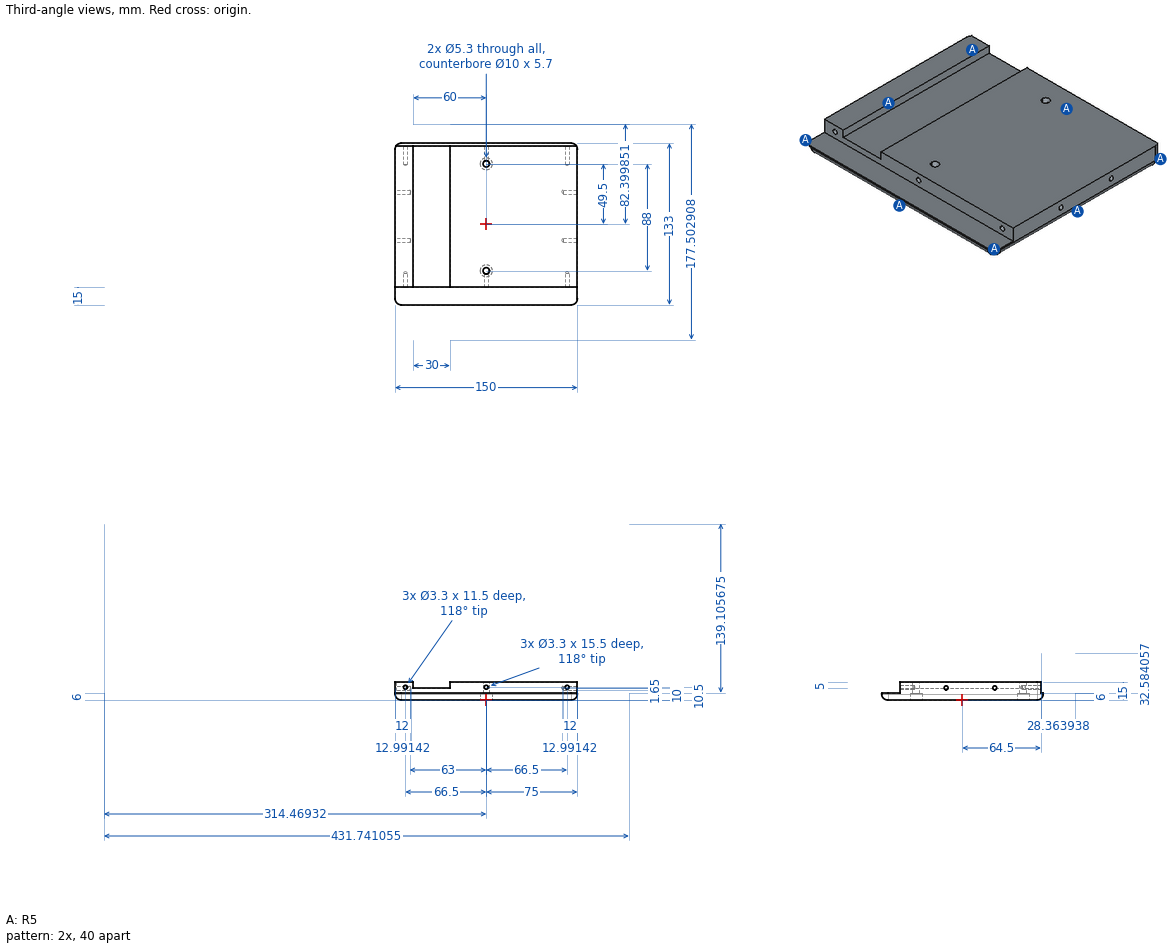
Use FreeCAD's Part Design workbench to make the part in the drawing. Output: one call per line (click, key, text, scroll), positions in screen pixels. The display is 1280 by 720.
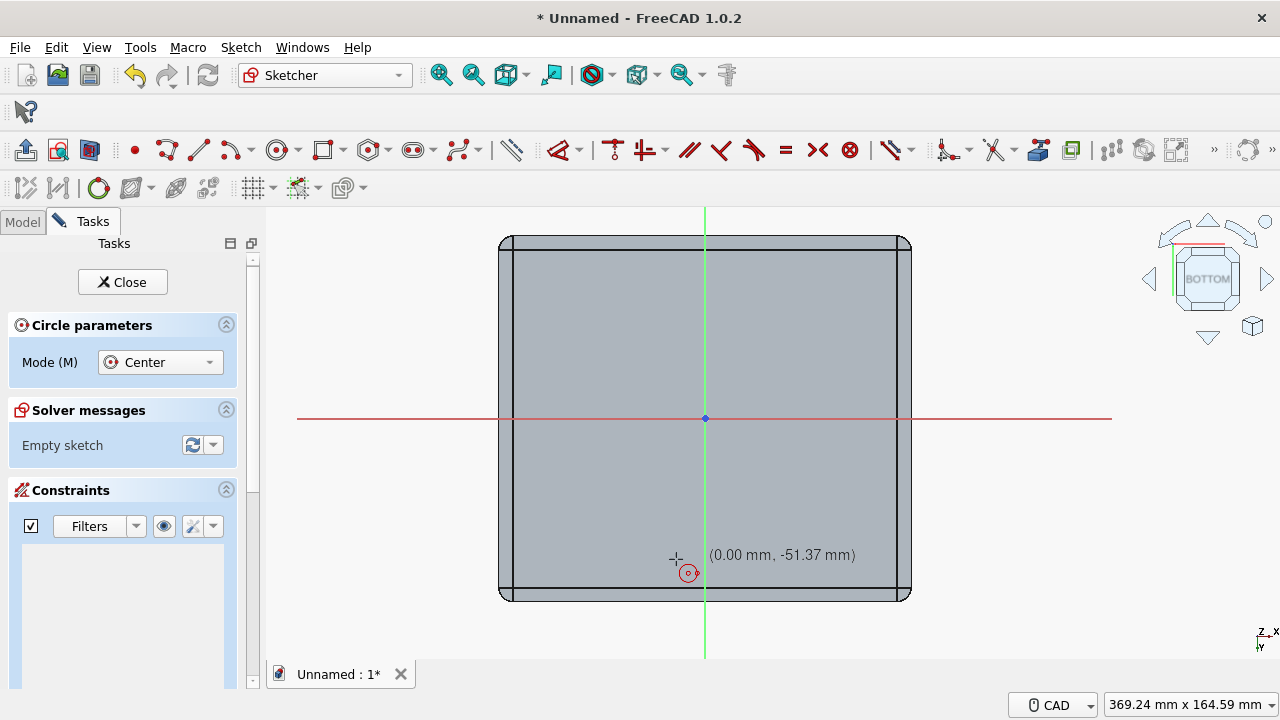
click(705, 555)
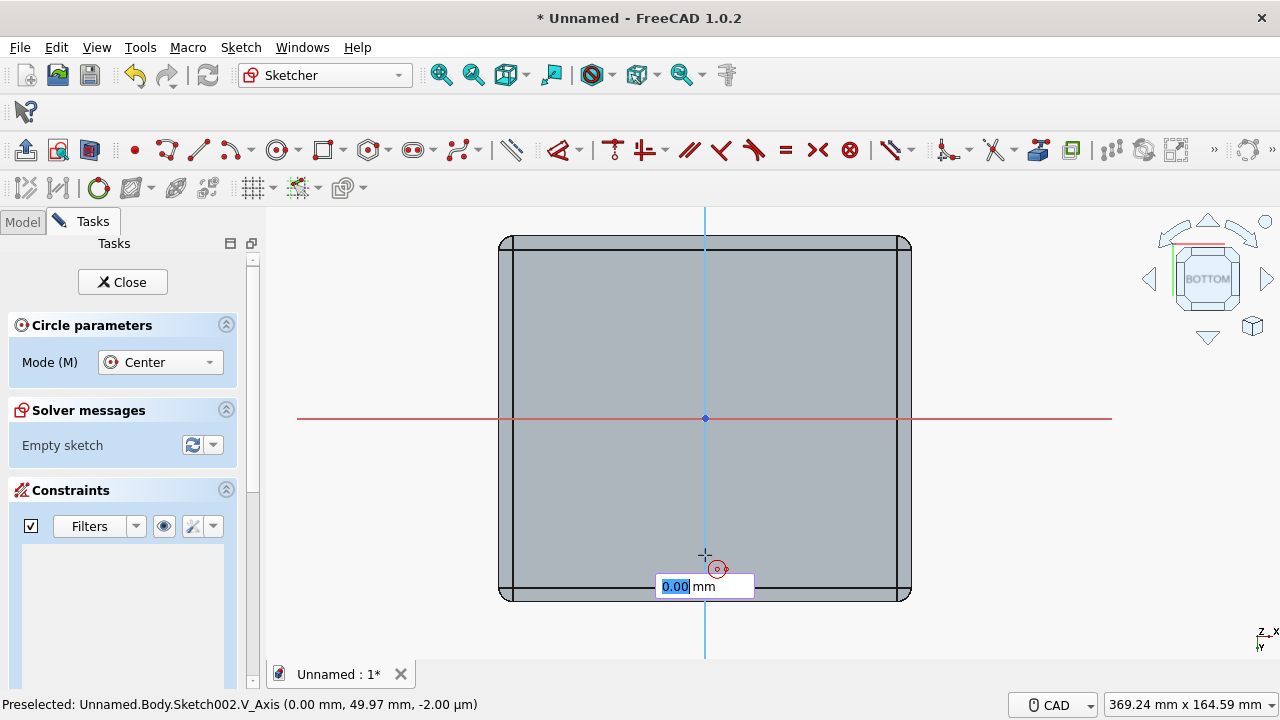
scroll(712, 552, up, 5)
move(711, 551)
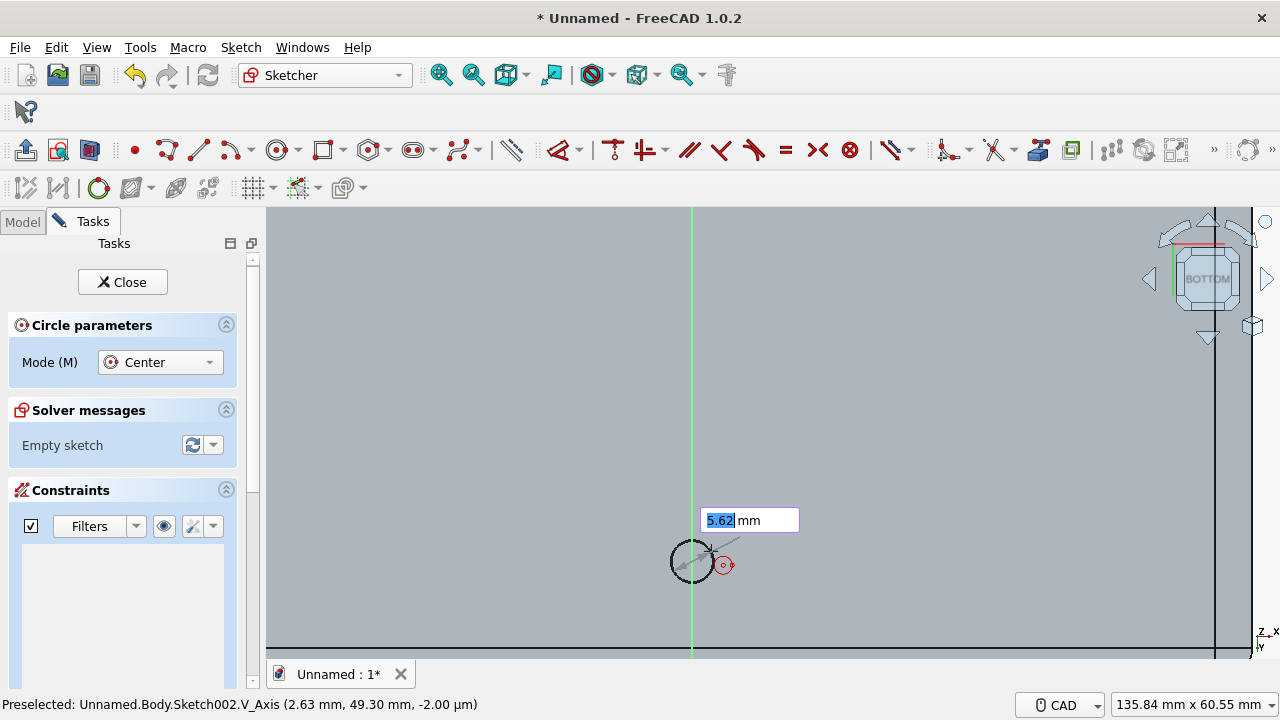
text(5.3)
key(Return)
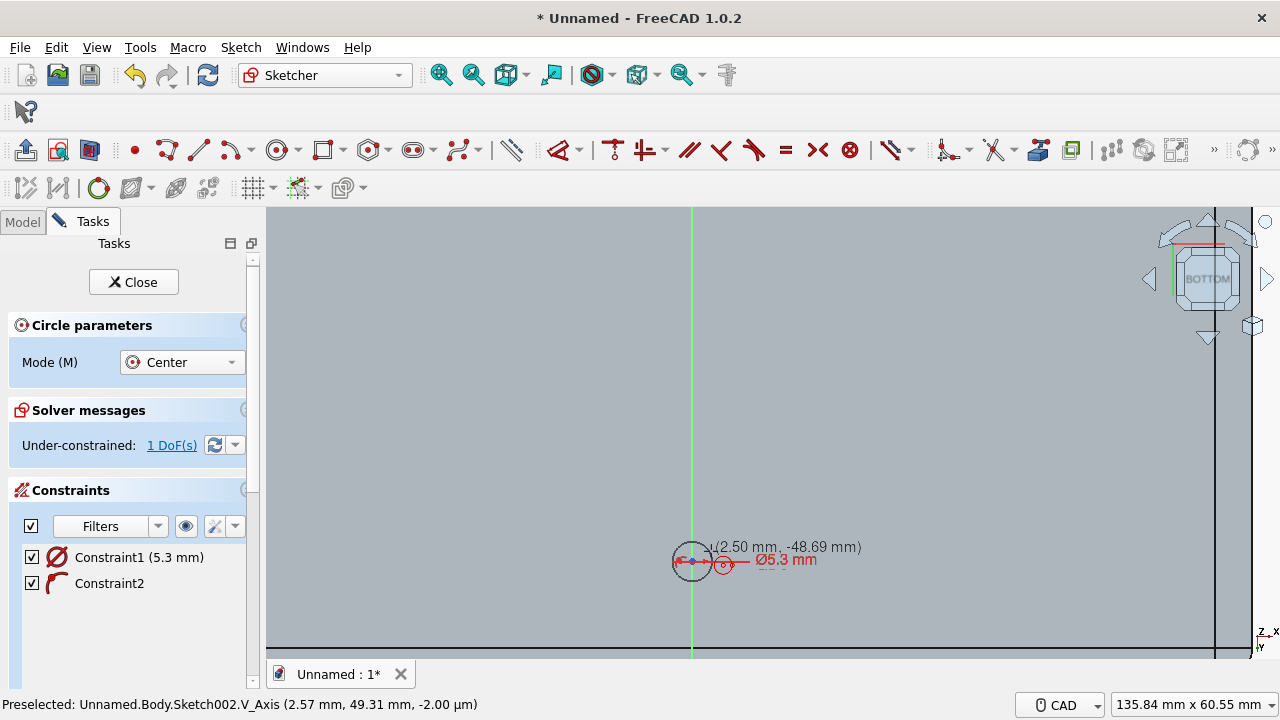
scroll(712, 551, down, 5)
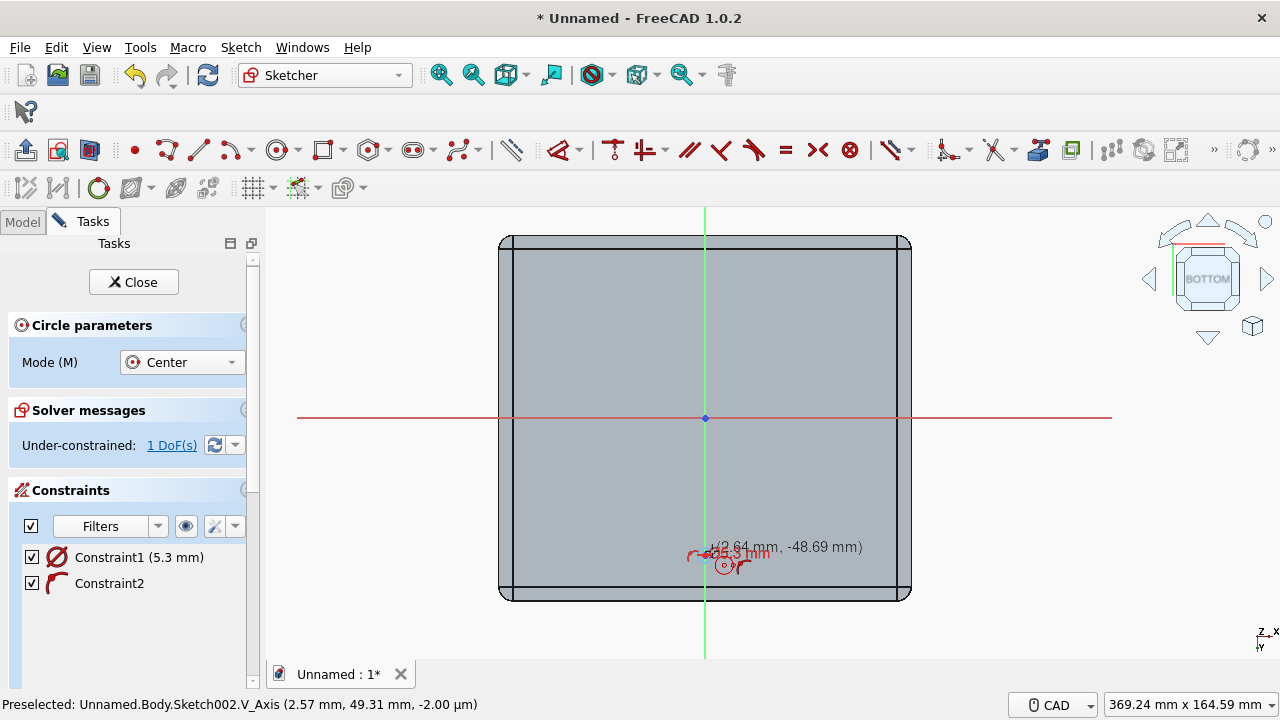
scroll(705, 312, up, 6)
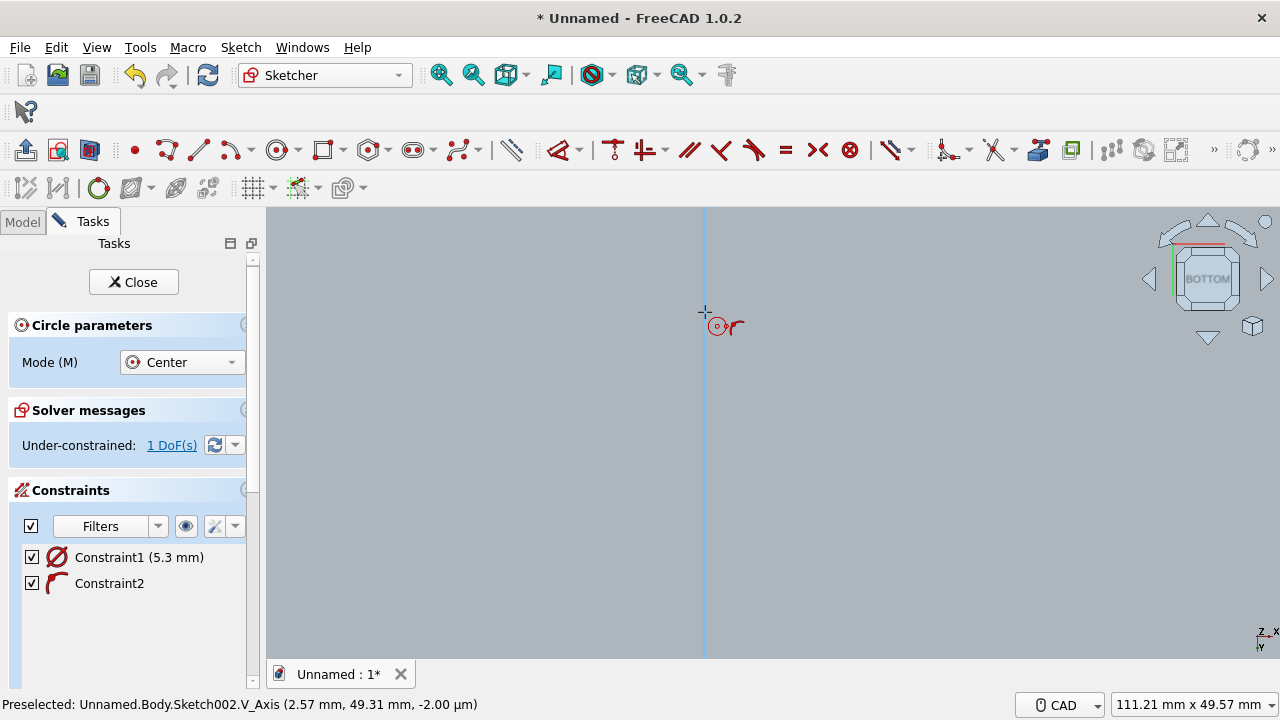
scroll(705, 312, down, 6)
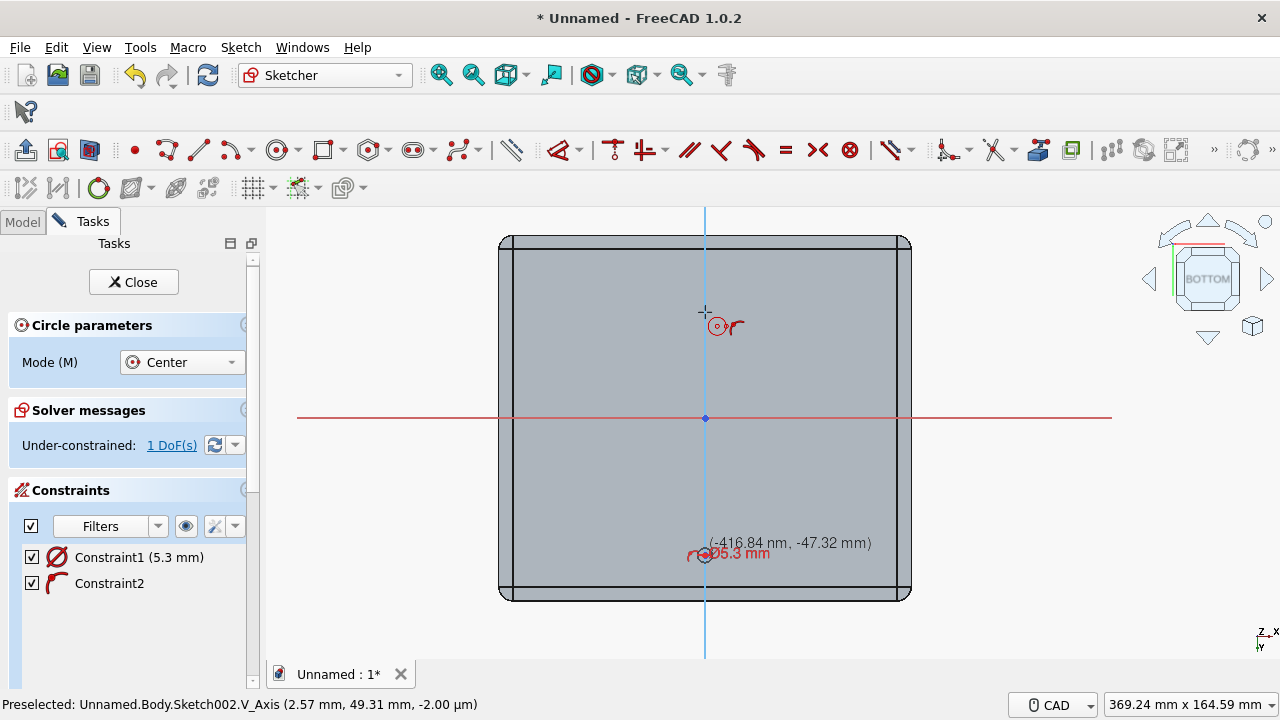
click(705, 312)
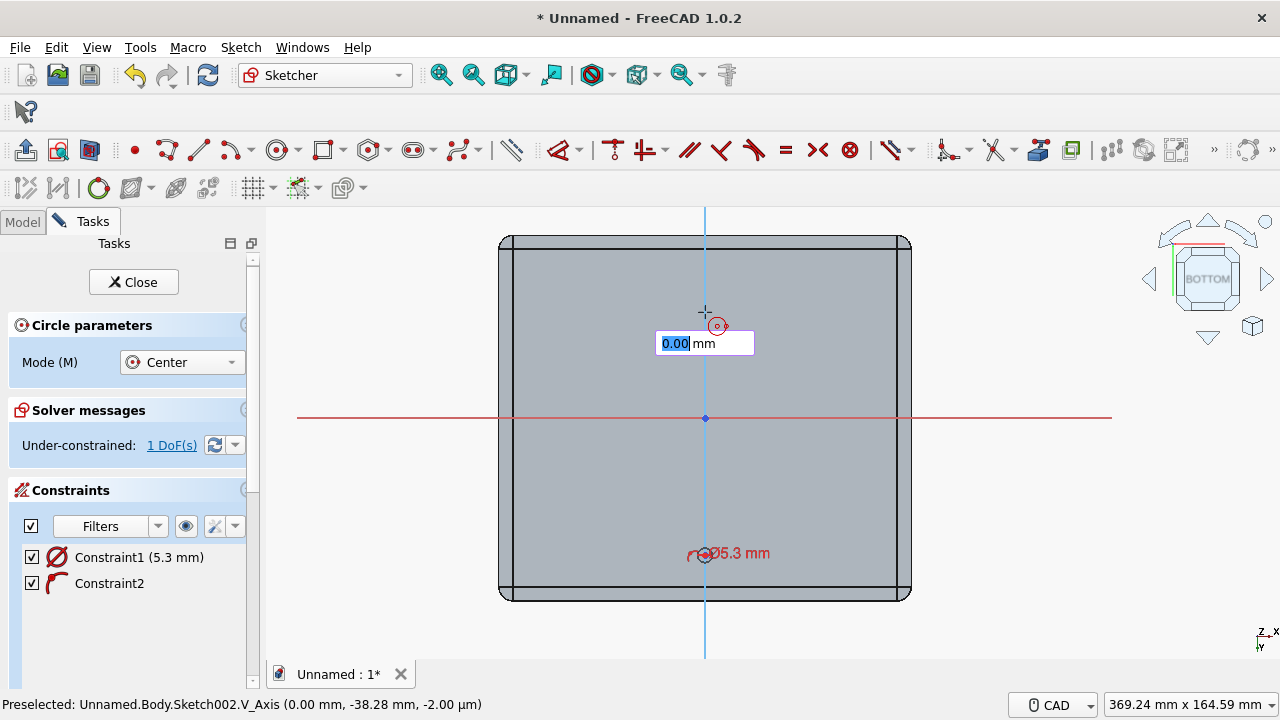
scroll(712, 310, up, 5)
move(711, 309)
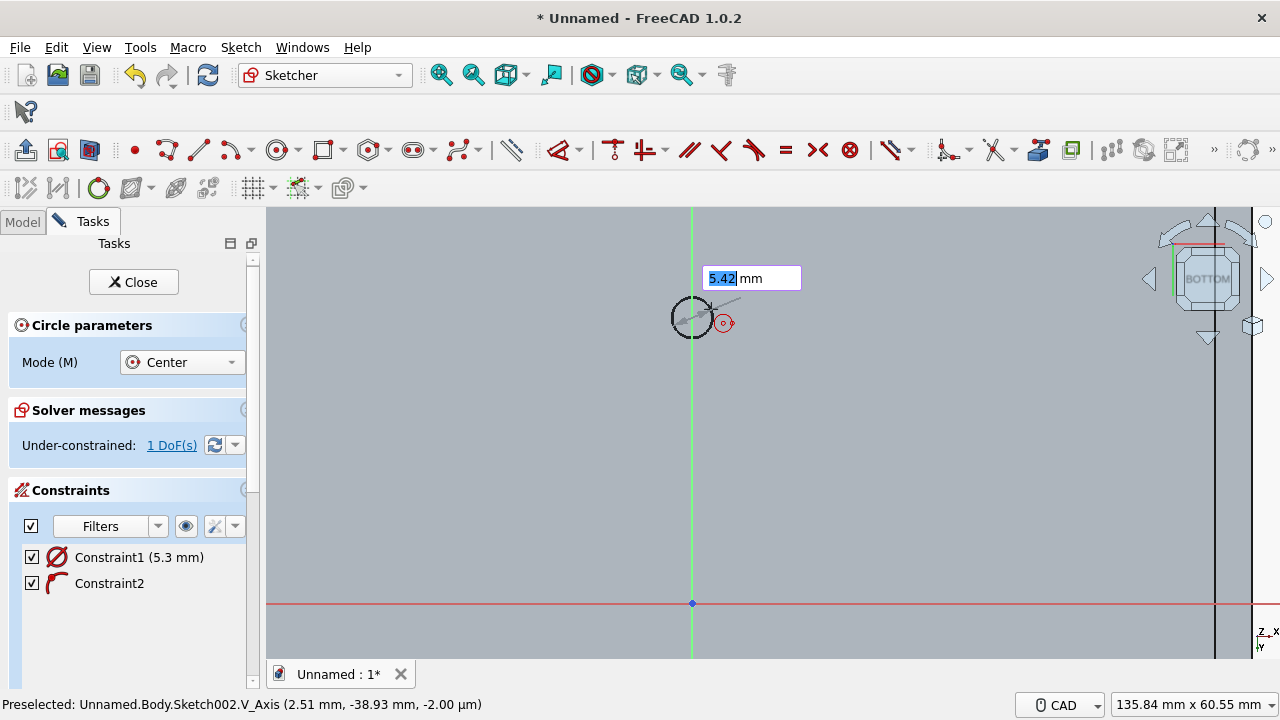
text(5.3)
key(Return)
key(Escape)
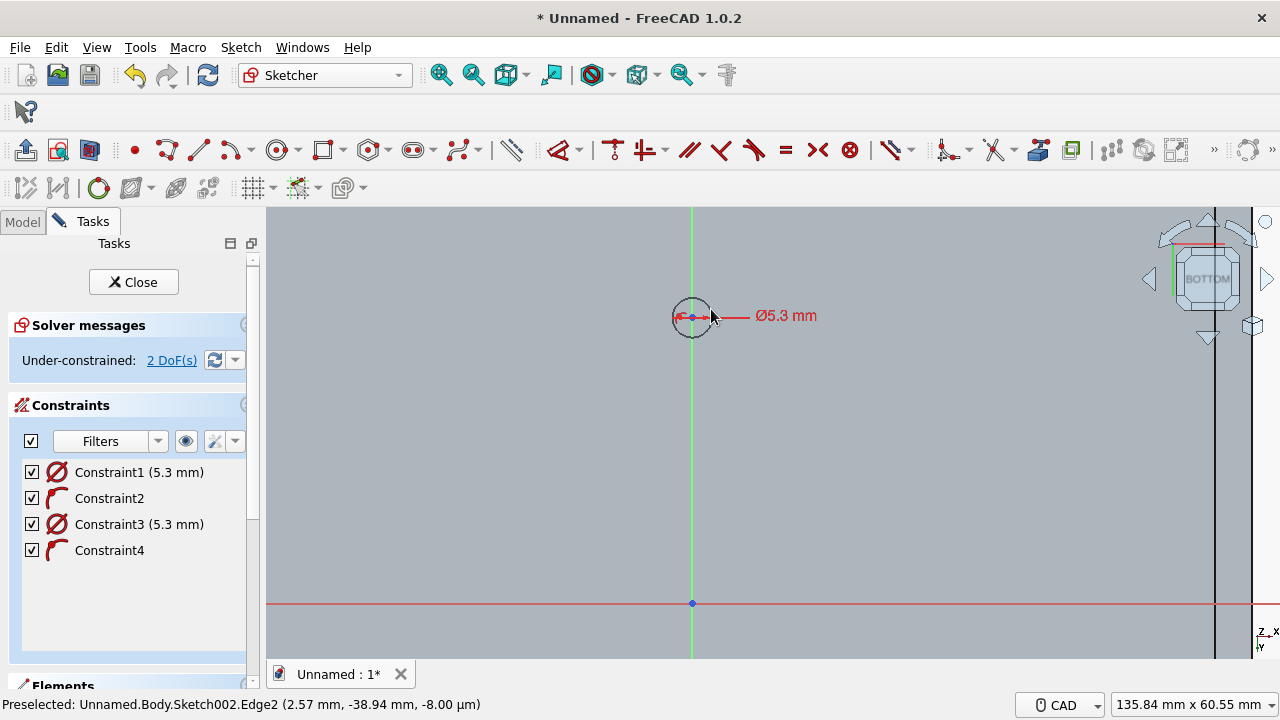
click(558, 150)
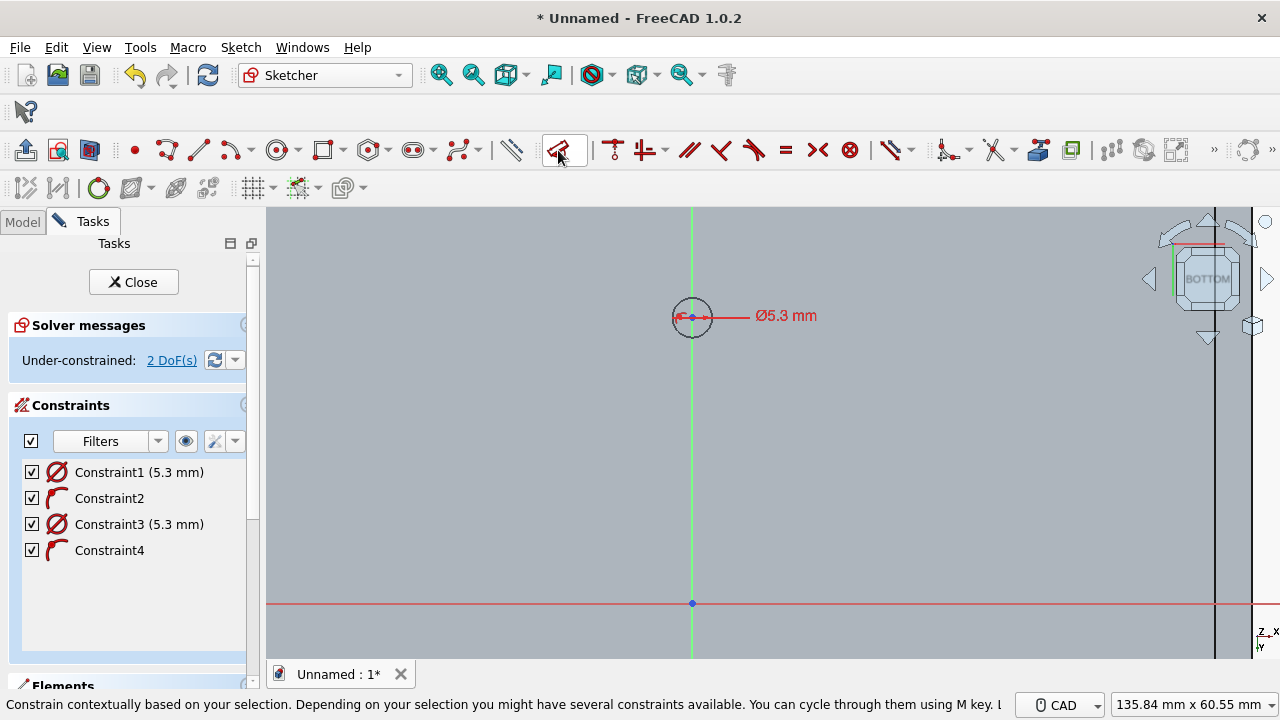
scroll(712, 310, down, 5)